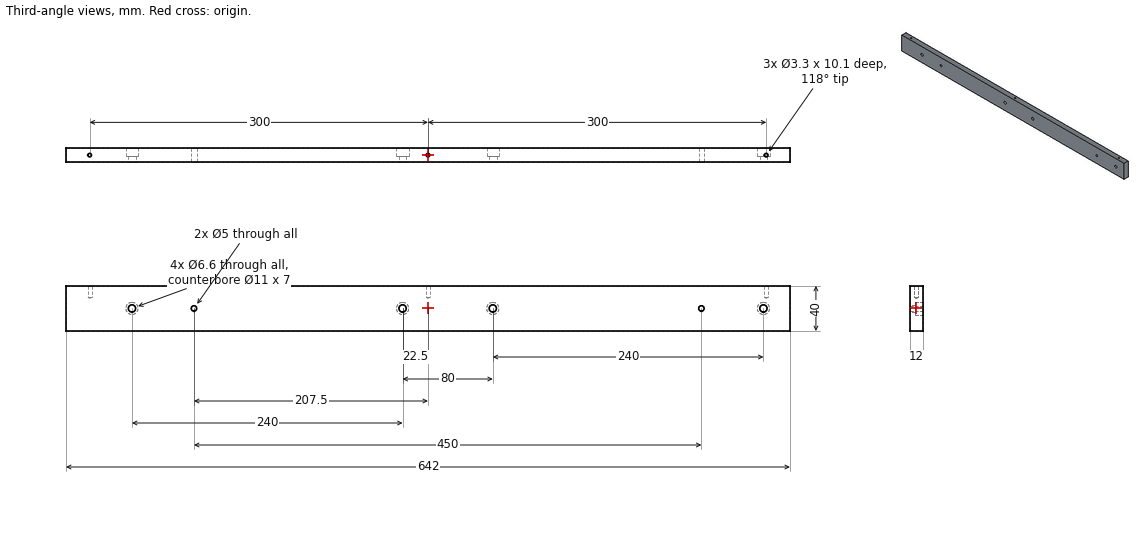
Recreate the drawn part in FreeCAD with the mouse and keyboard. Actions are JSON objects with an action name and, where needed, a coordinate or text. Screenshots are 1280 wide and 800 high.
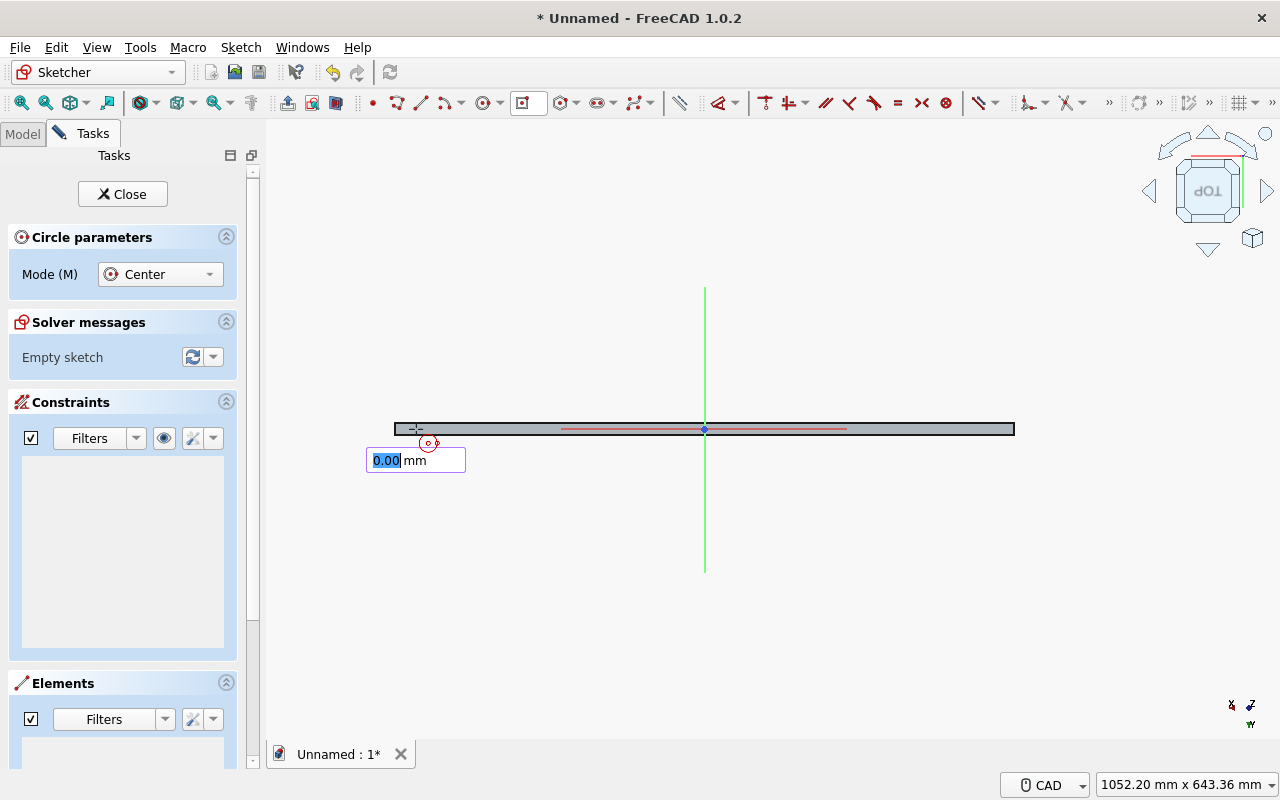
{"action": "scroll", "coordinate": [415, 431], "scroll_direction": "up", "scroll_amount": 12}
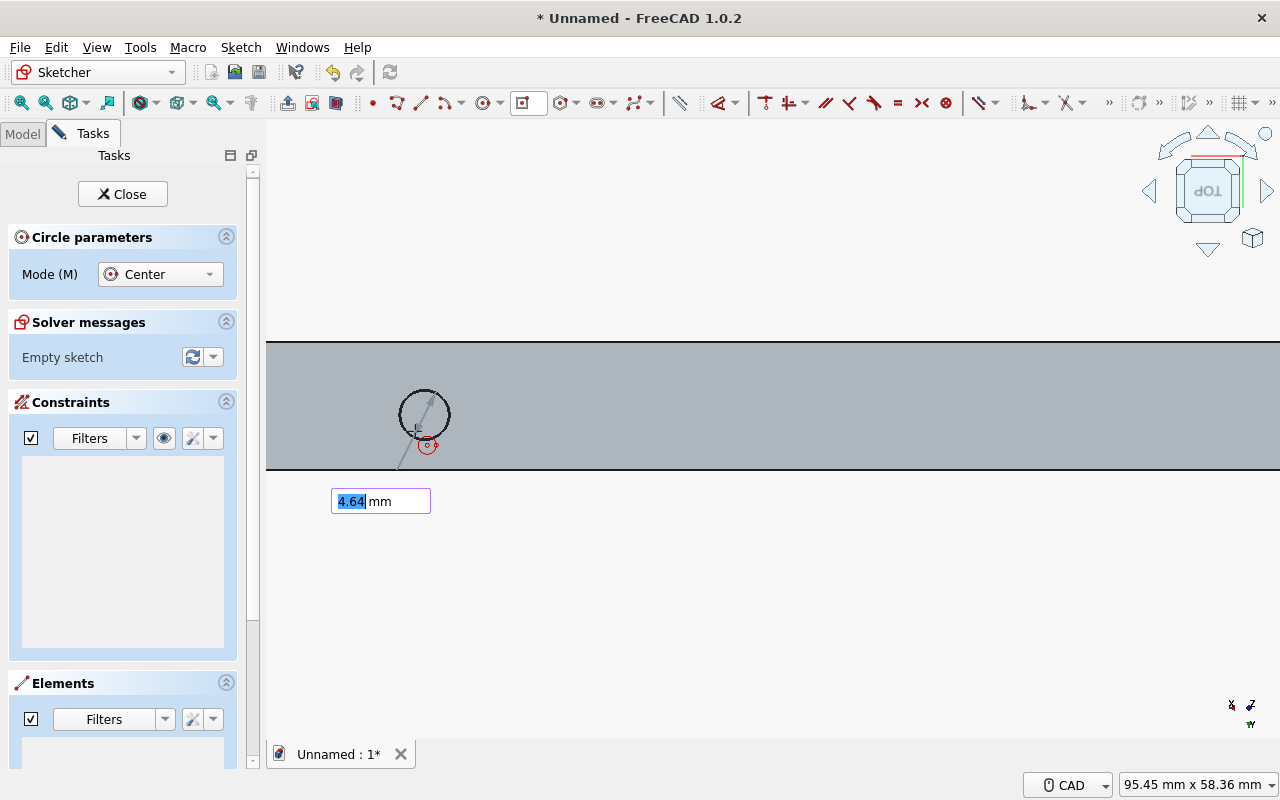
{"action": "left_click", "coordinate": [414, 423]}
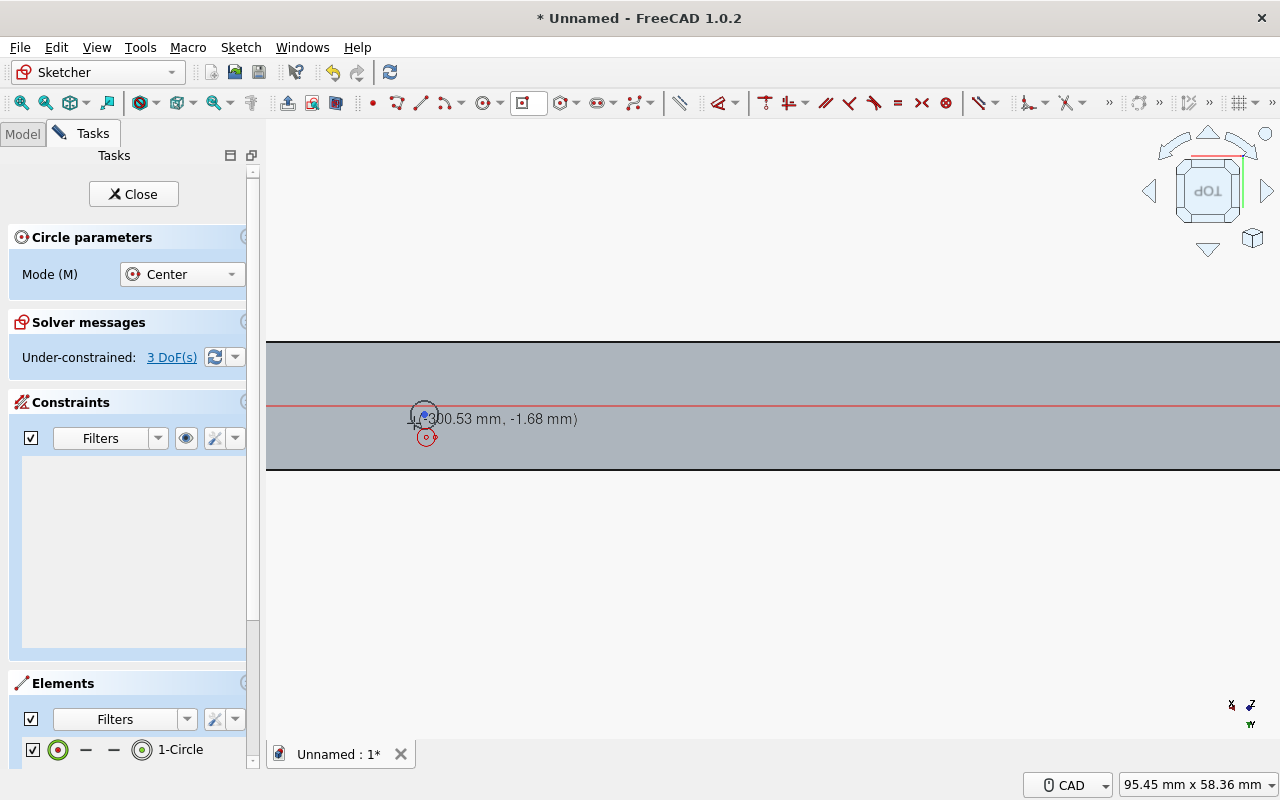
{"action": "scroll", "coordinate": [415, 431], "scroll_direction": "down", "scroll_amount": 12}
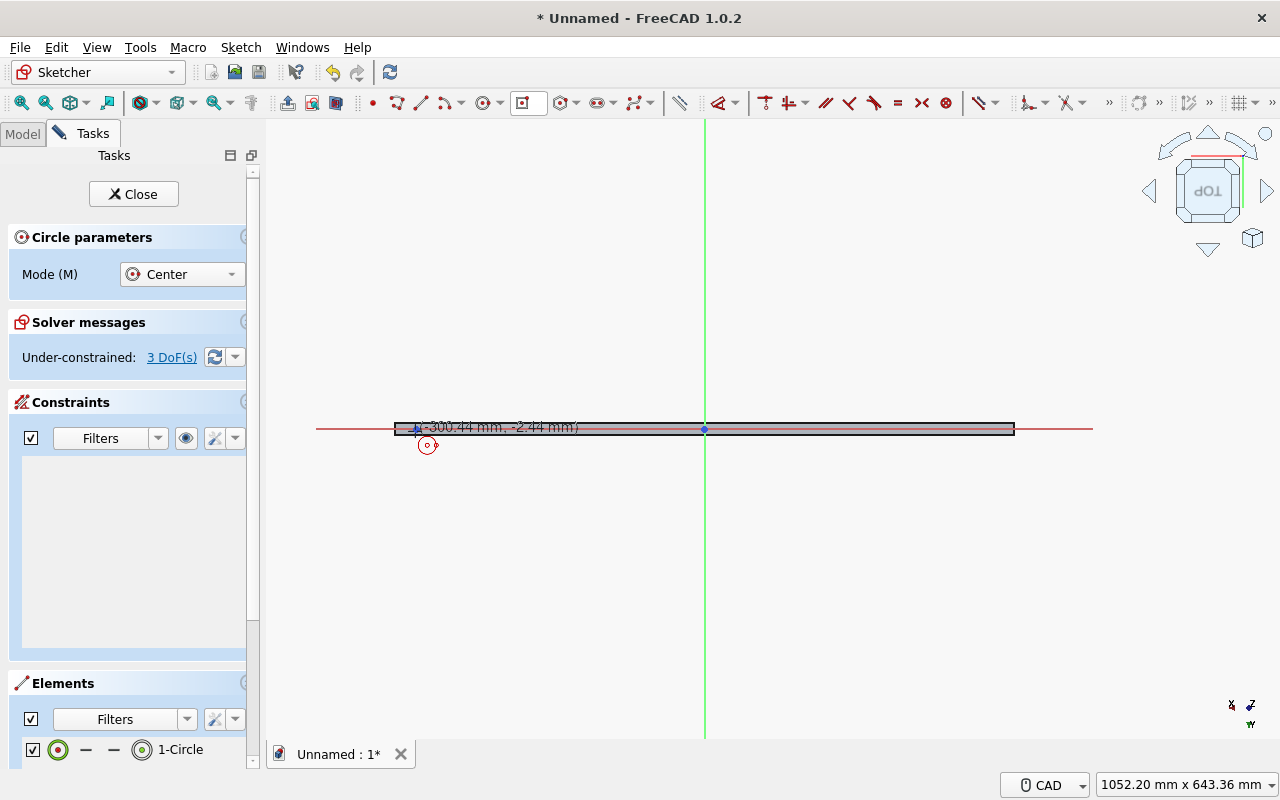
{"action": "scroll", "coordinate": [705, 429], "scroll_direction": "up", "scroll_amount": 14}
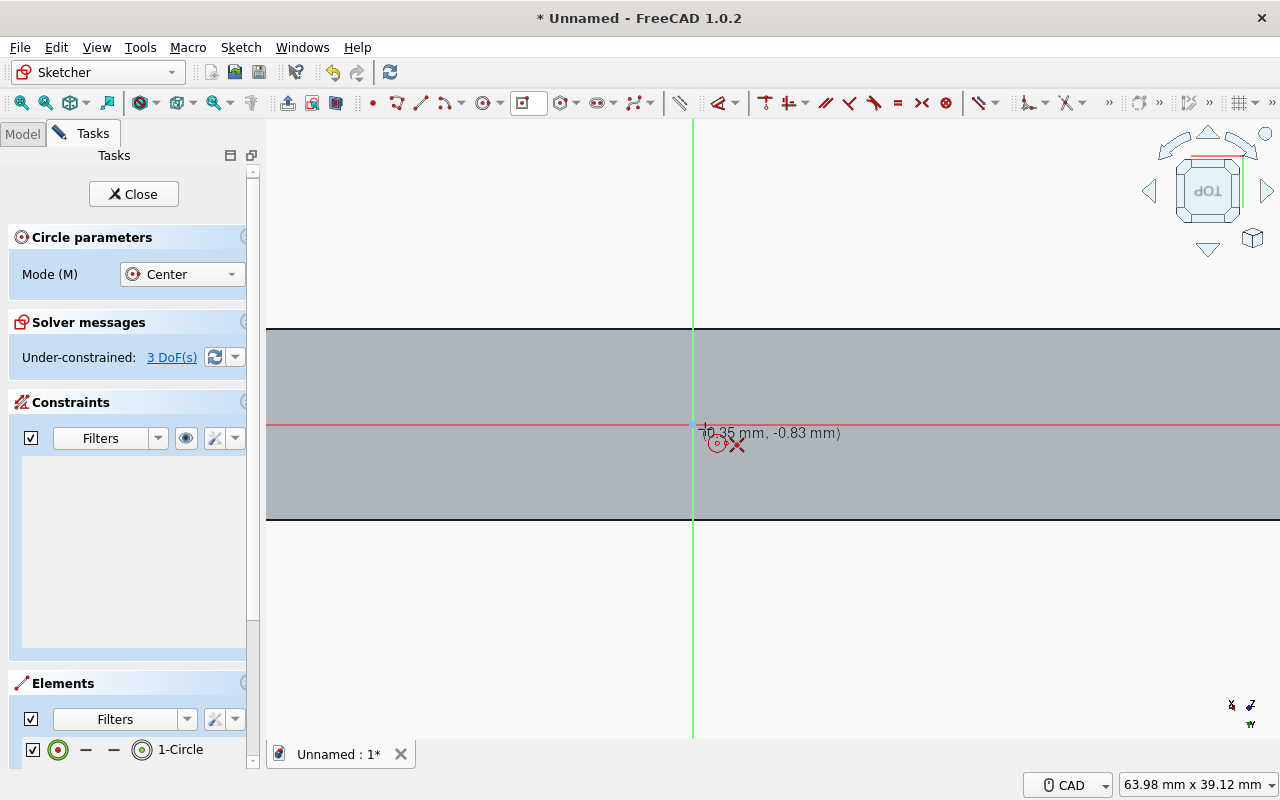
{"action": "scroll", "coordinate": [705, 429], "scroll_direction": "down", "scroll_amount": 14}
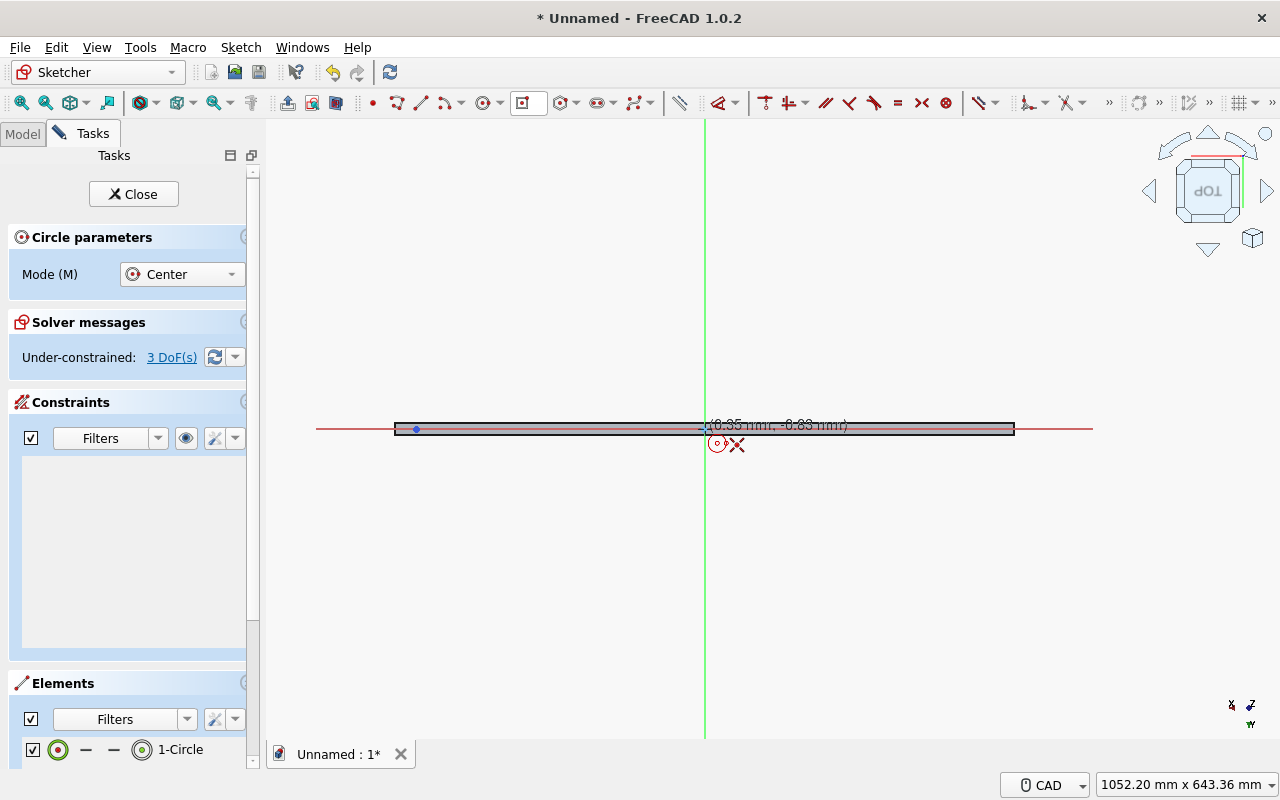
{"action": "left_click", "coordinate": [705, 429]}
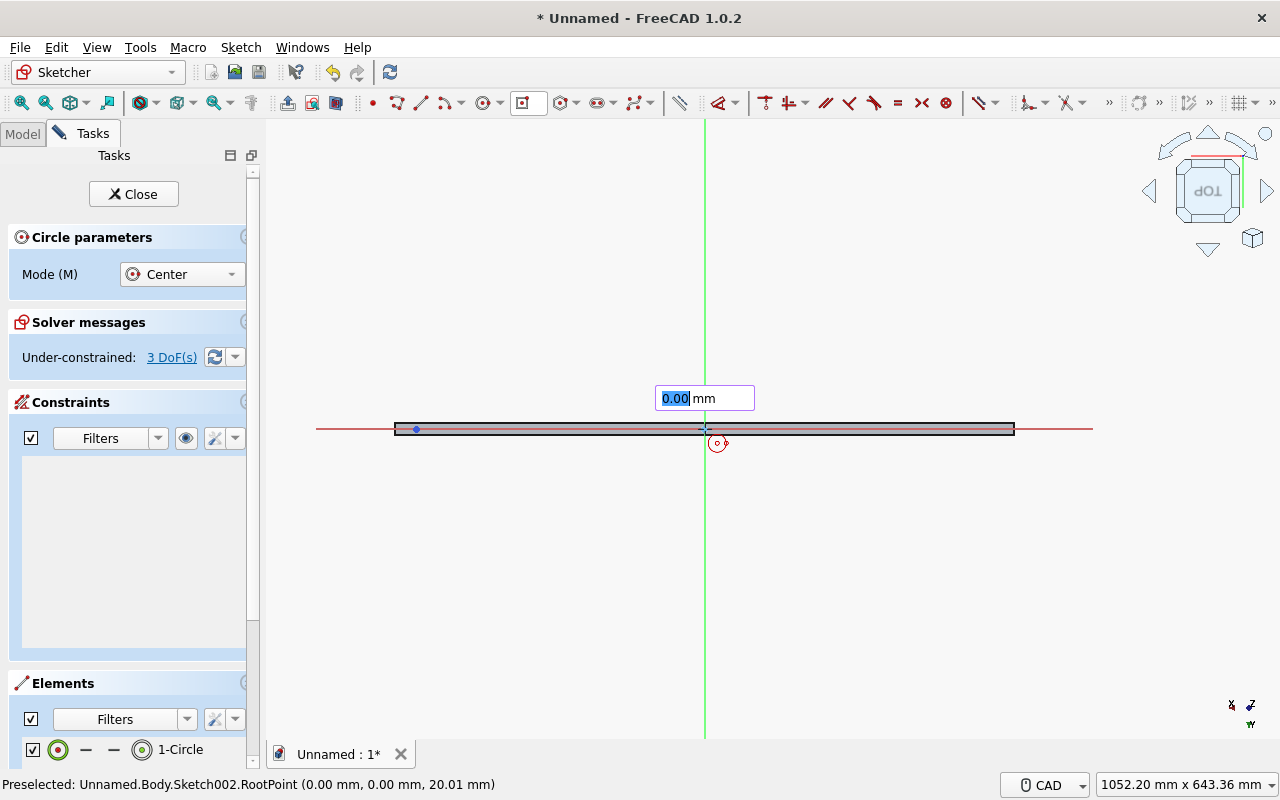
{"action": "scroll", "coordinate": [706, 428], "scroll_direction": "up", "scroll_amount": 14}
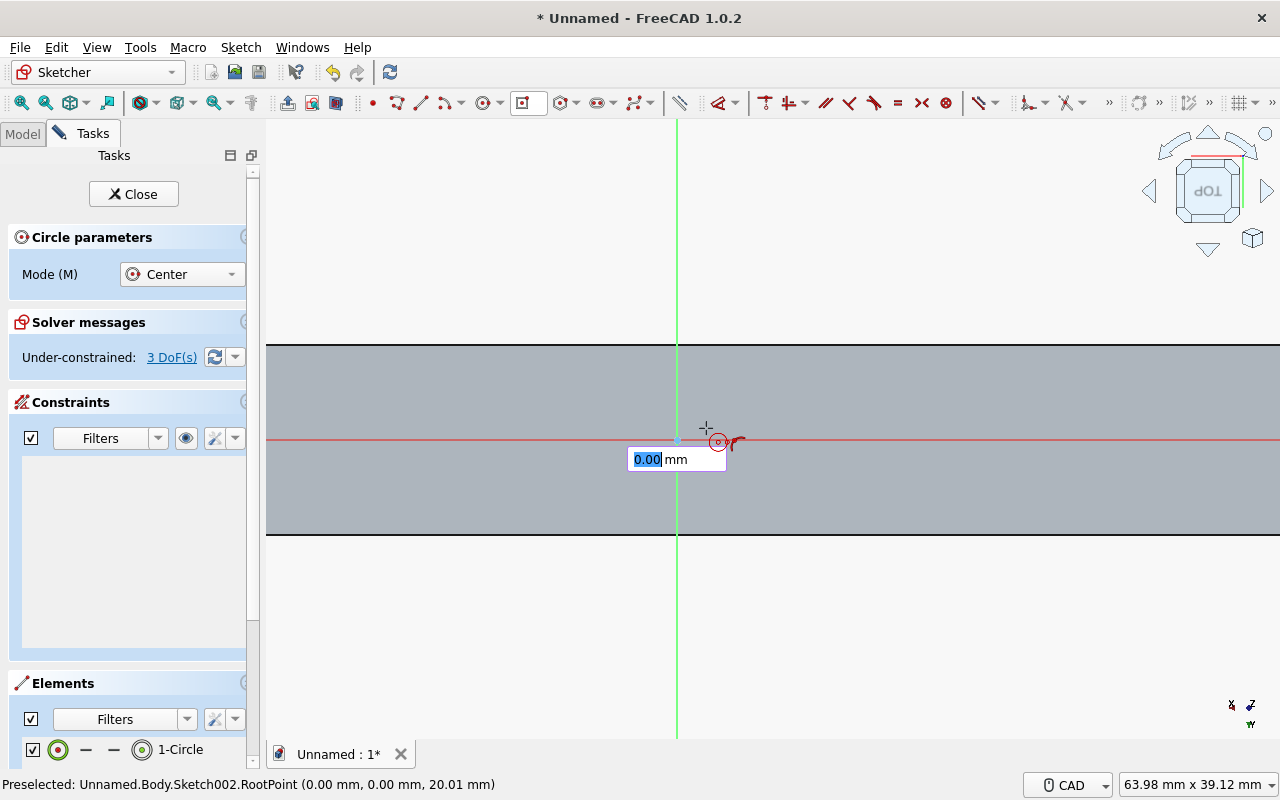
{"action": "left_click", "coordinate": [696, 422]}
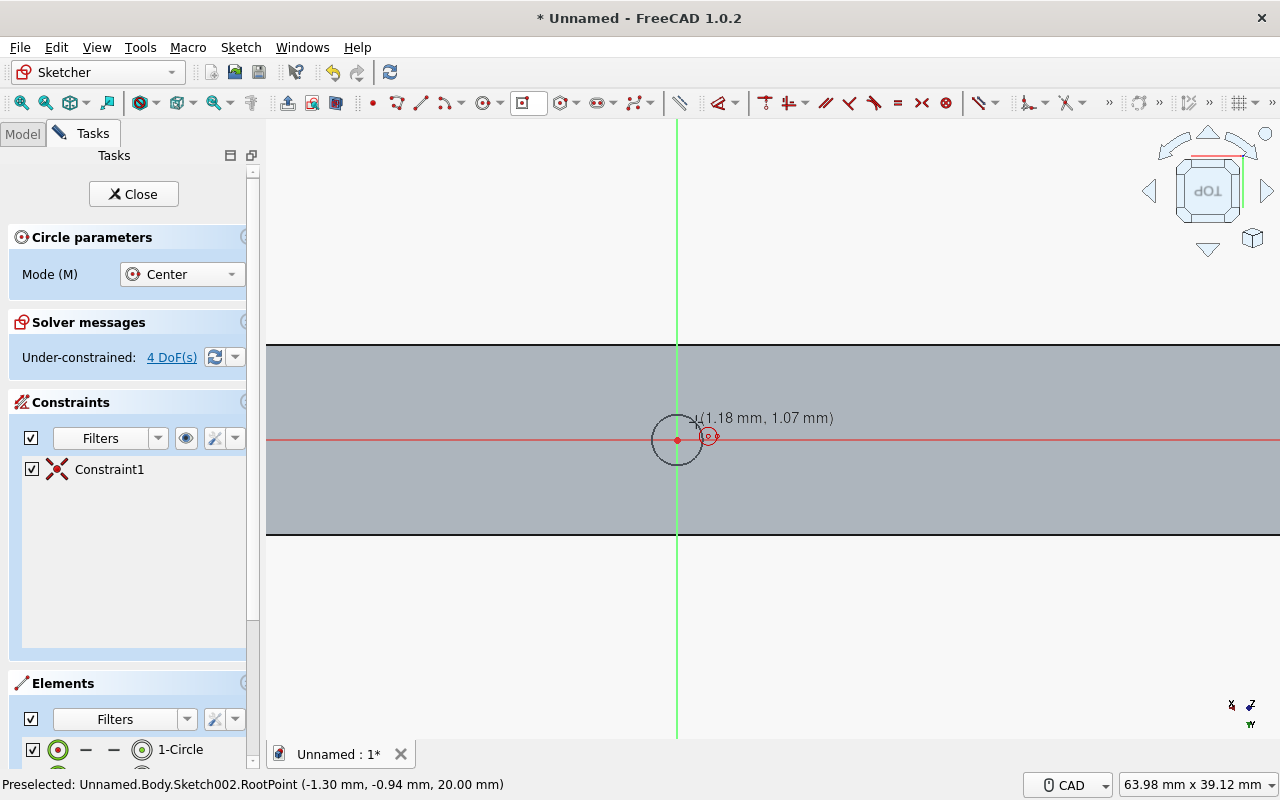
{"action": "scroll", "coordinate": [706, 428], "scroll_direction": "down", "scroll_amount": 14}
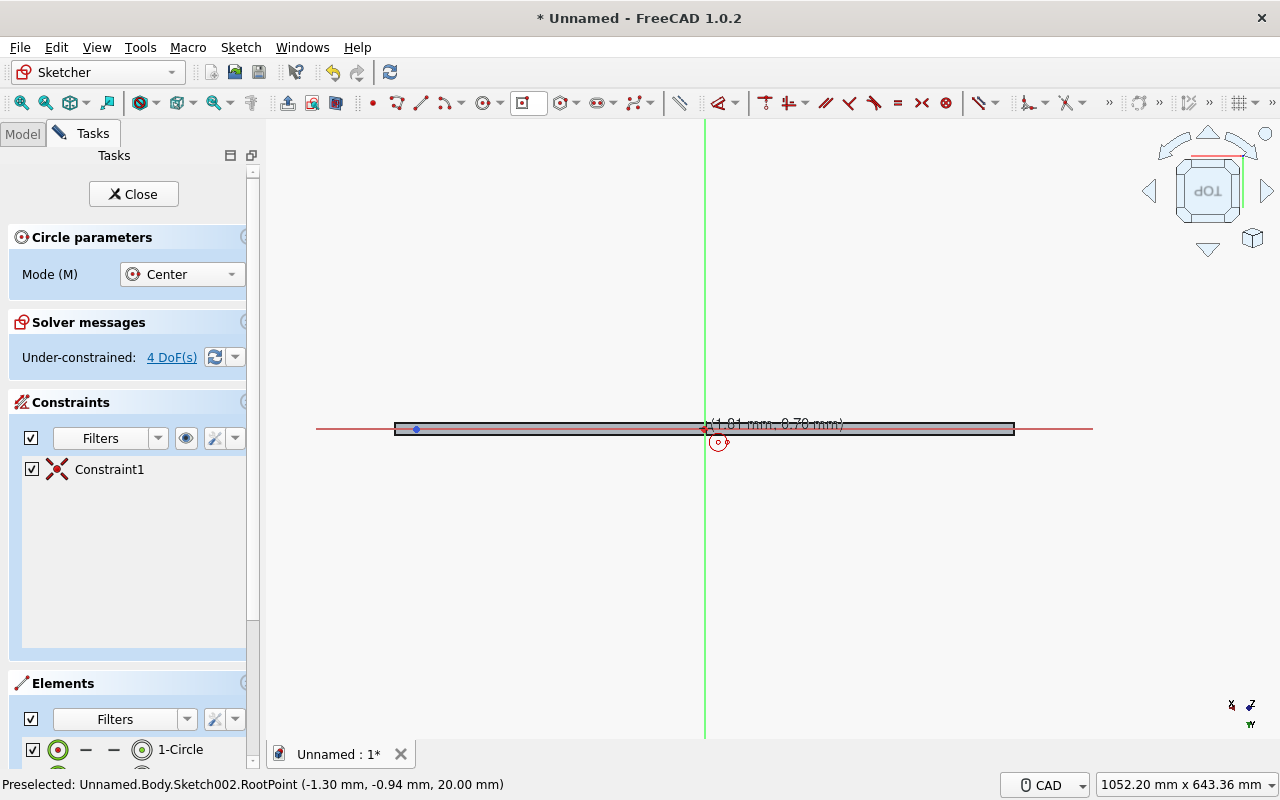
{"action": "scroll", "coordinate": [994, 429], "scroll_direction": "up", "scroll_amount": 14}